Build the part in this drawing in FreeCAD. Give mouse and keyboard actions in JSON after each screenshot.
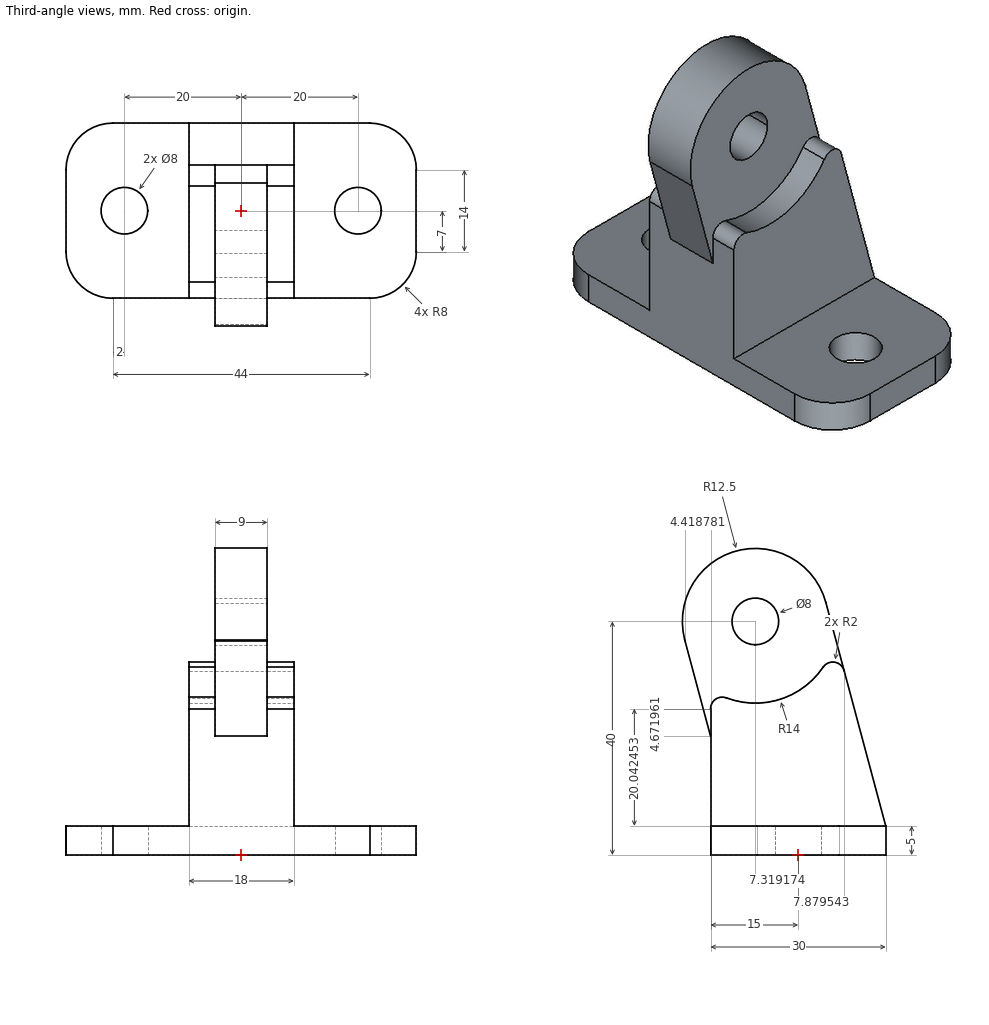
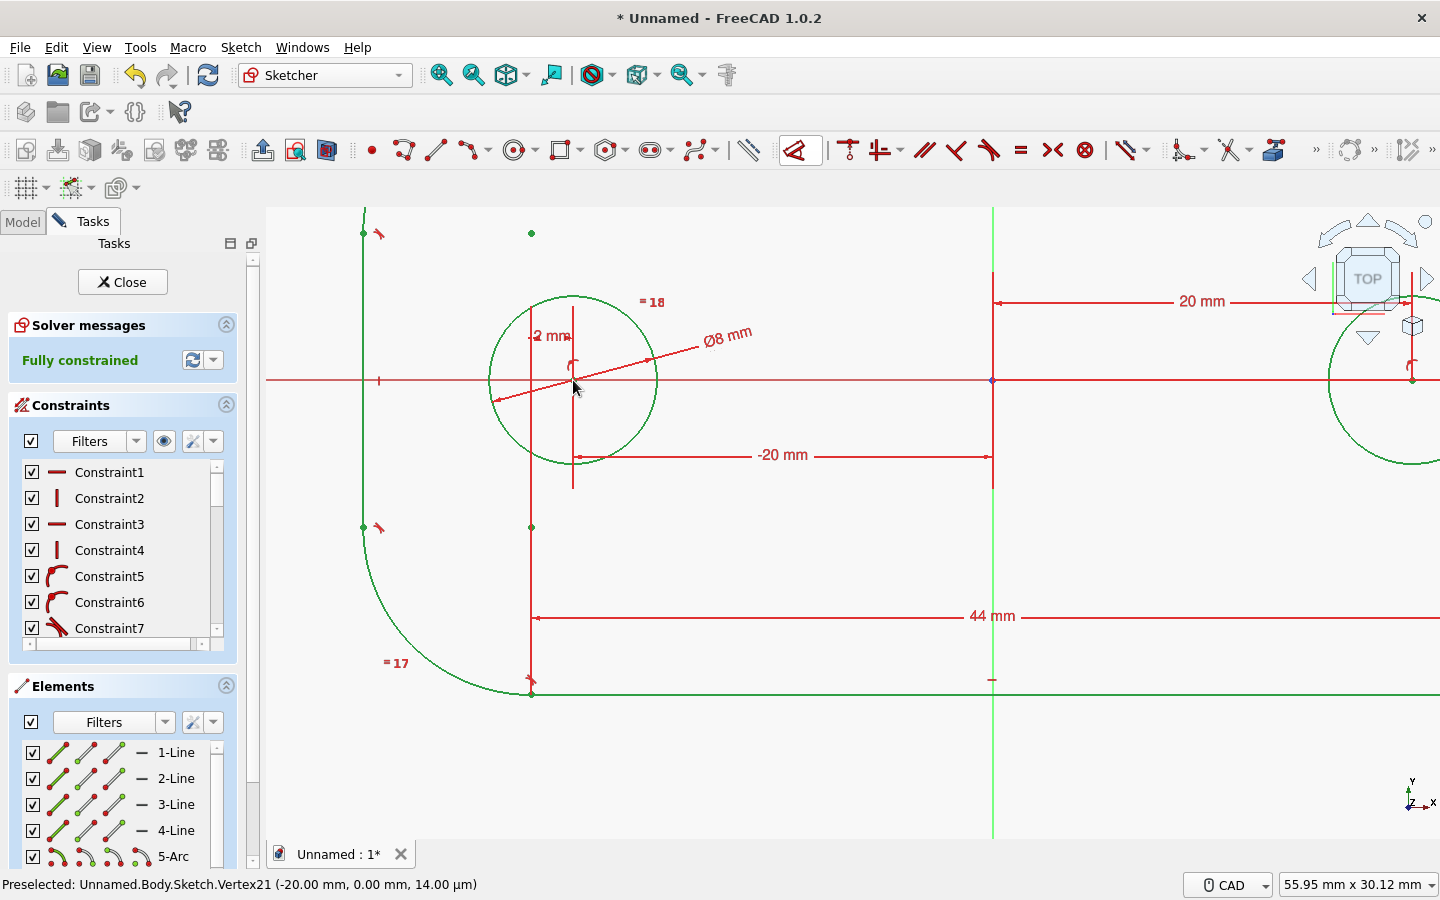
{"action": "left_click", "coordinate": [123, 282]}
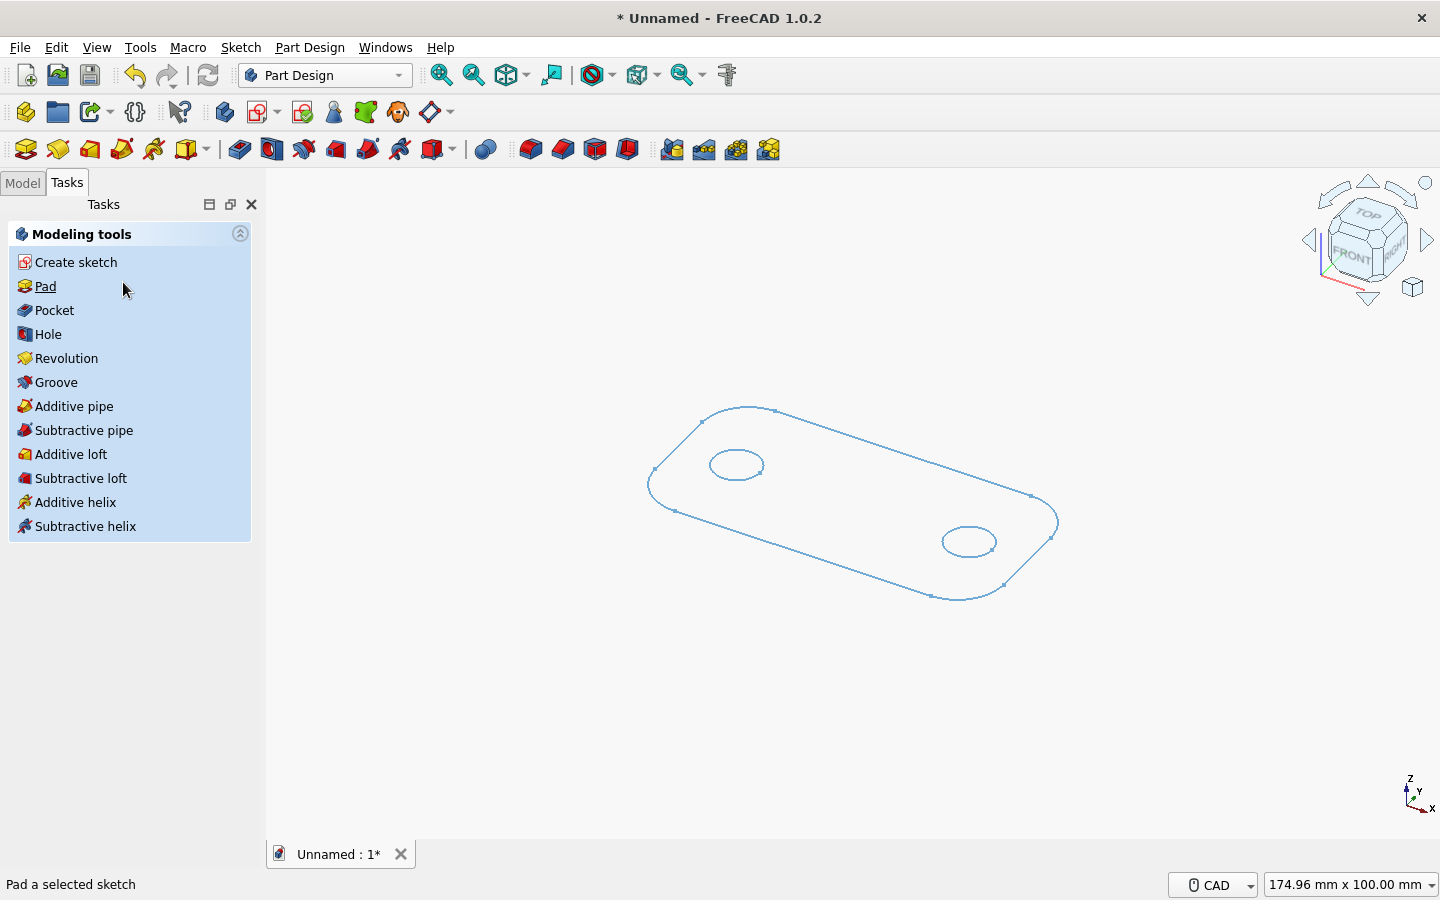
{"action": "left_click", "coordinate": [26, 150]}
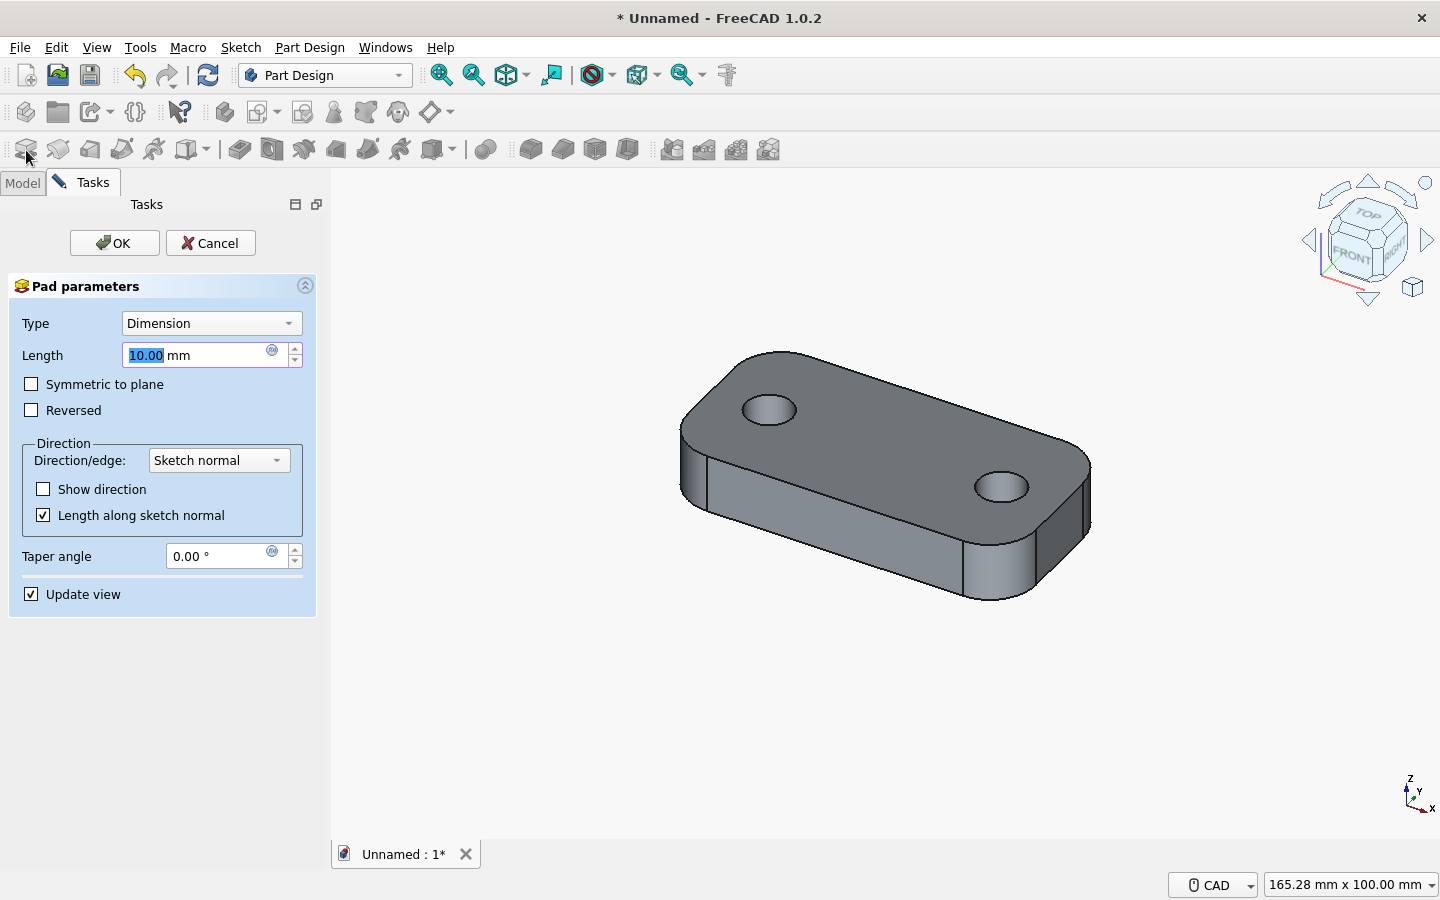
{"action": "type", "text": "5"}
{"action": "key", "text": "Tab"}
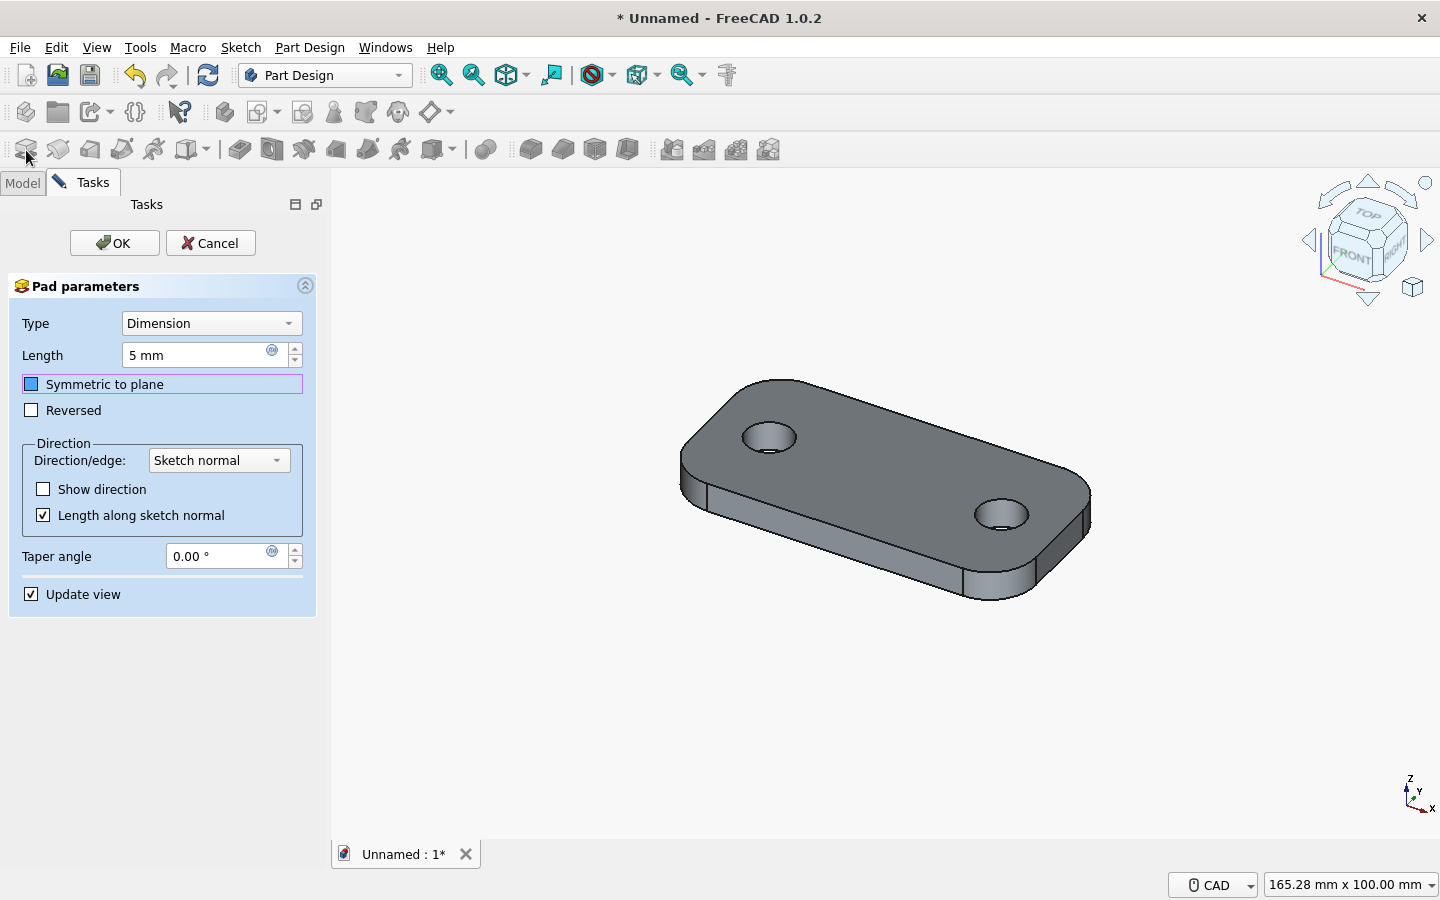
{"action": "left_click", "coordinate": [115, 243]}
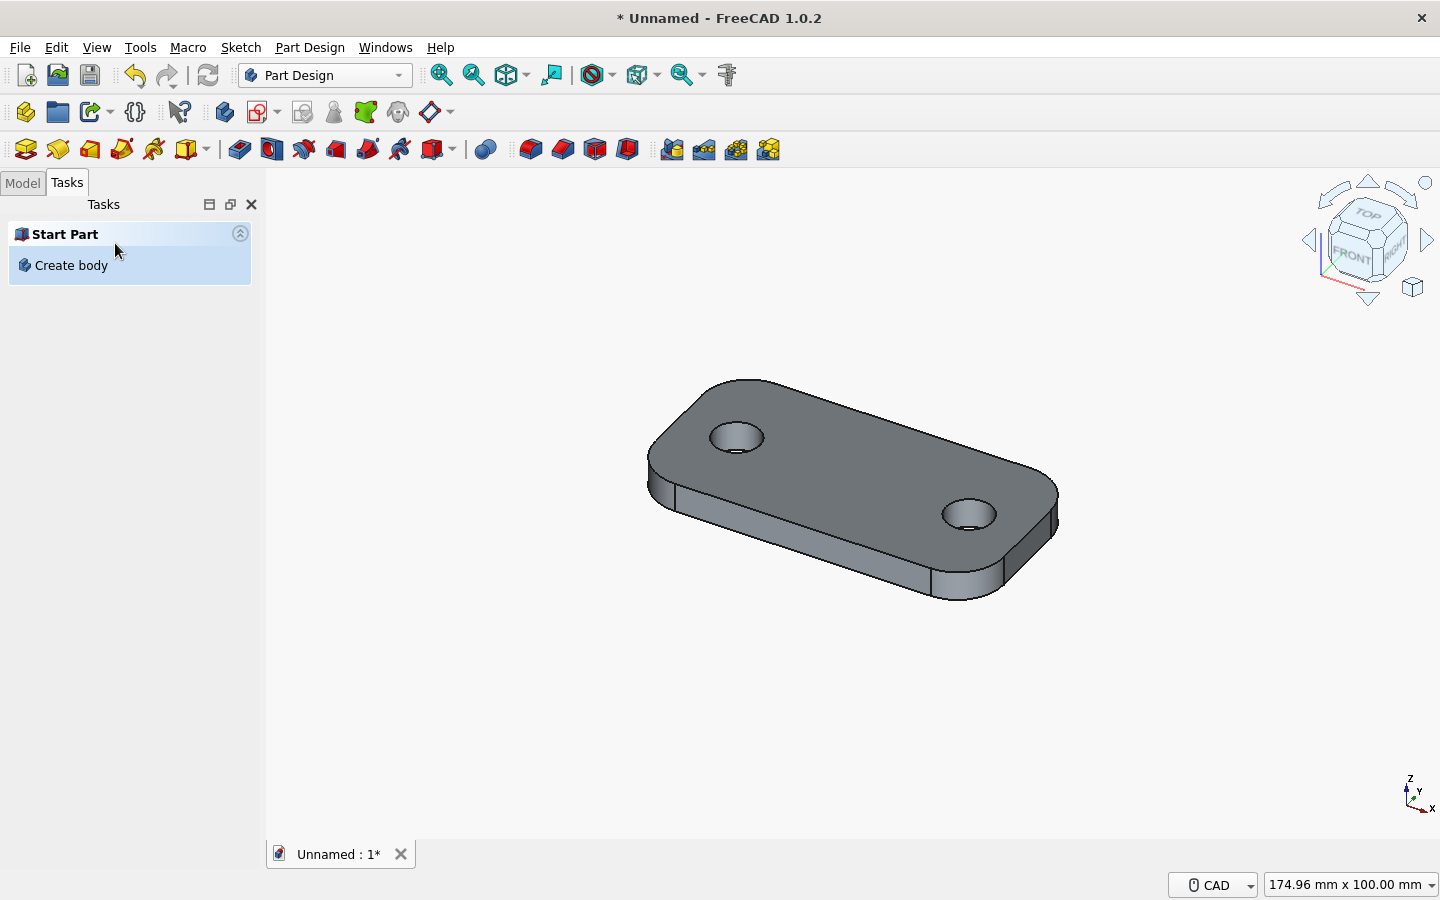
{"action": "key", "text": "v f"}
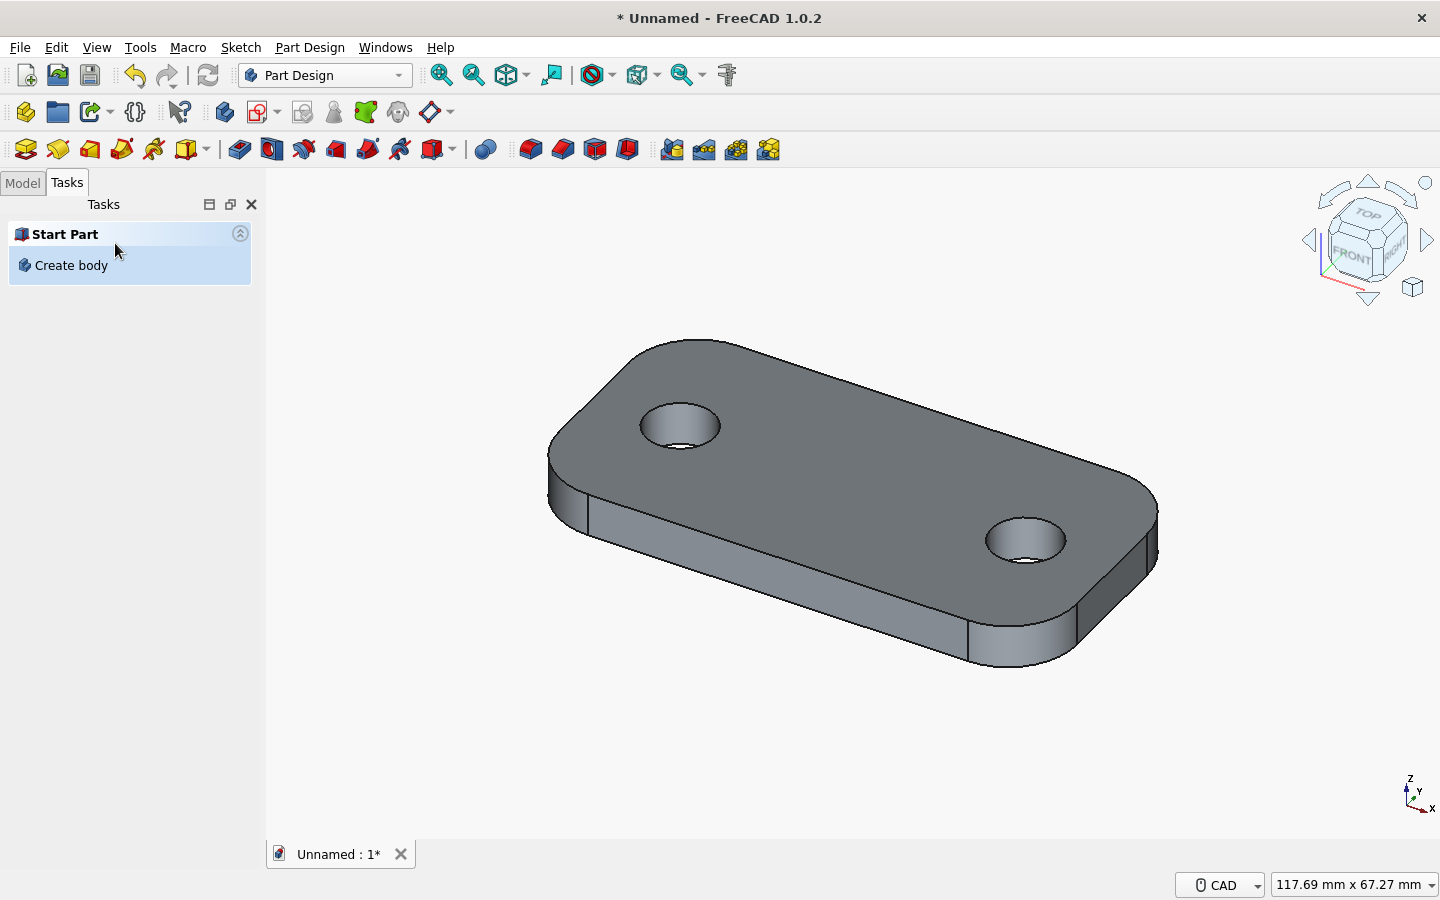
{"action": "left_click", "coordinate": [226, 112]}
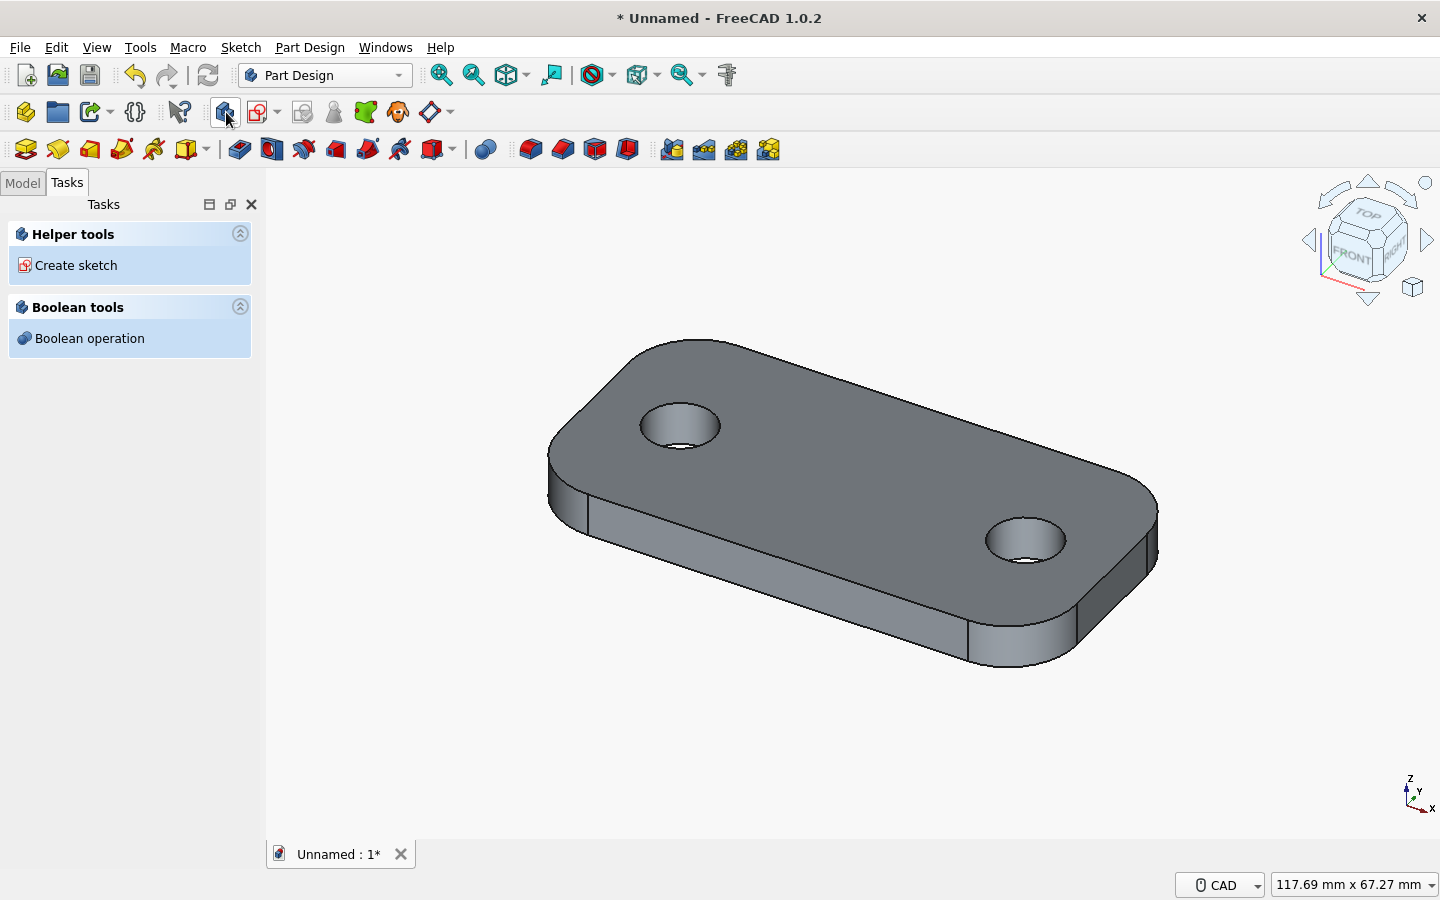
{"action": "left_click", "coordinate": [306, 799]}